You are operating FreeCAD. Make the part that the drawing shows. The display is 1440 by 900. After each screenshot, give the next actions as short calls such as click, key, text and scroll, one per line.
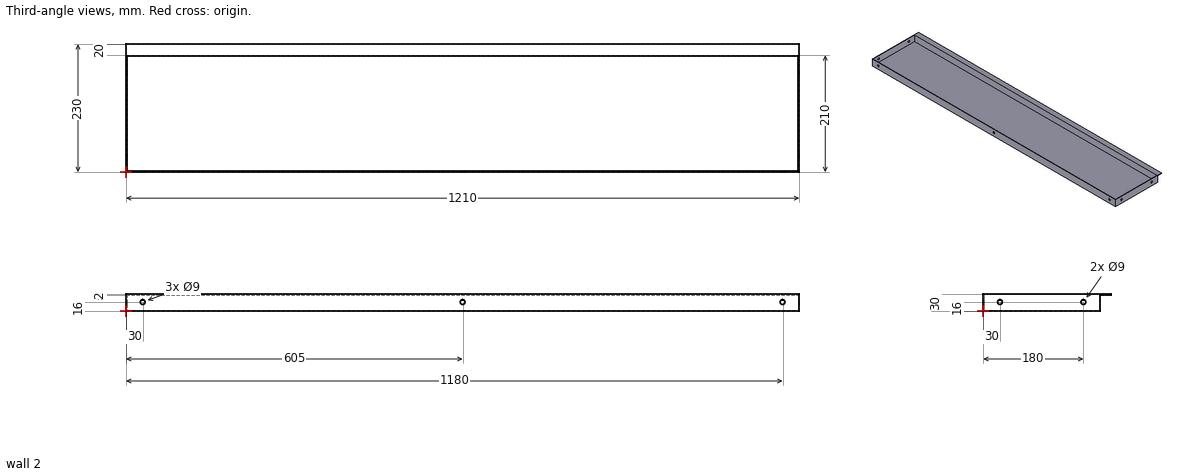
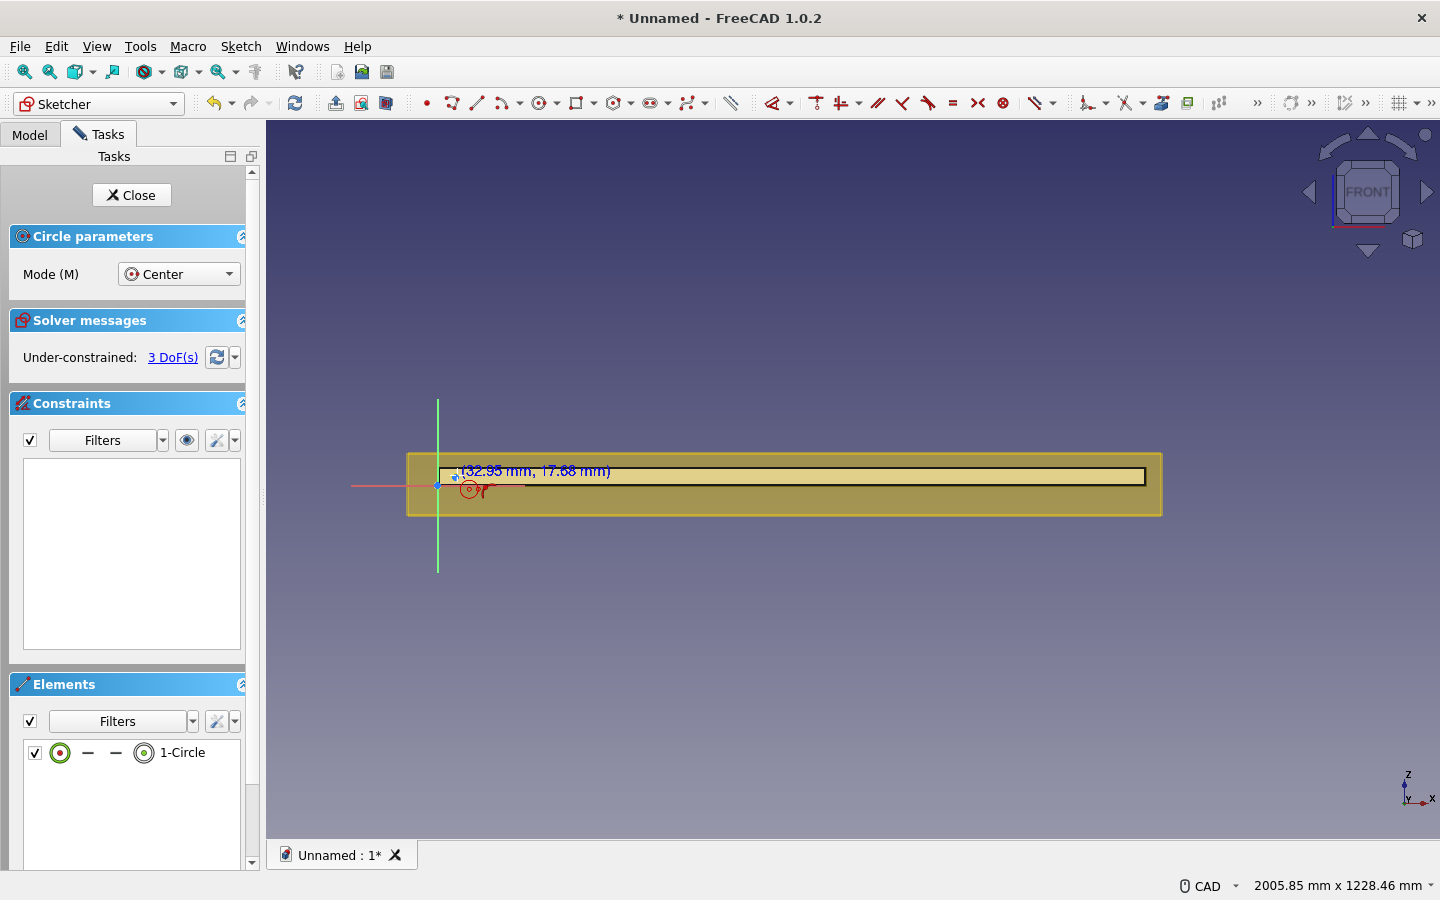
scroll(1128, 477, up, 11)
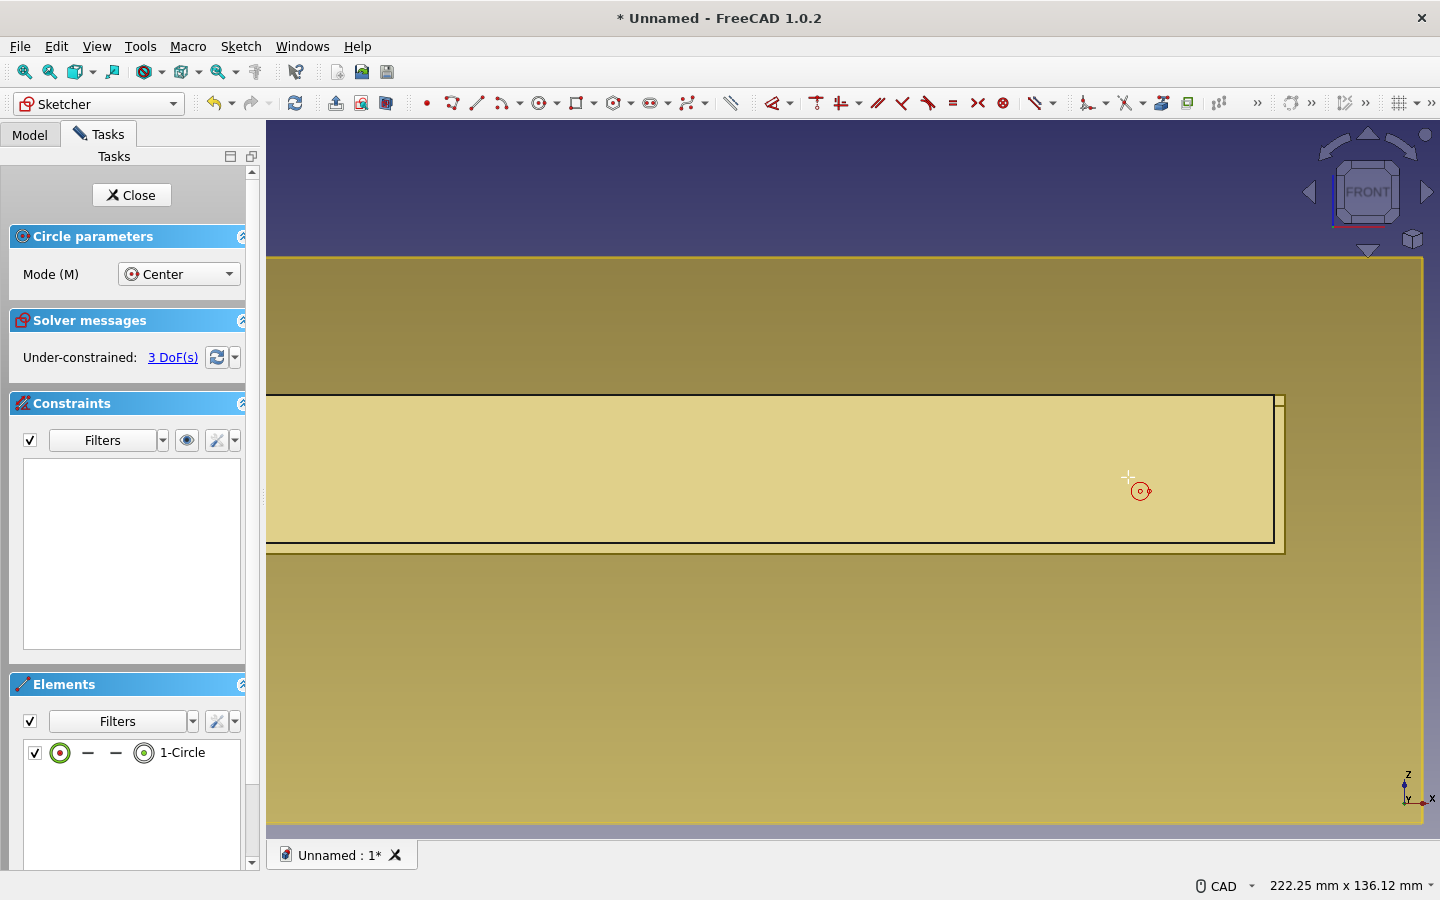
scroll(1129, 477, down, 11)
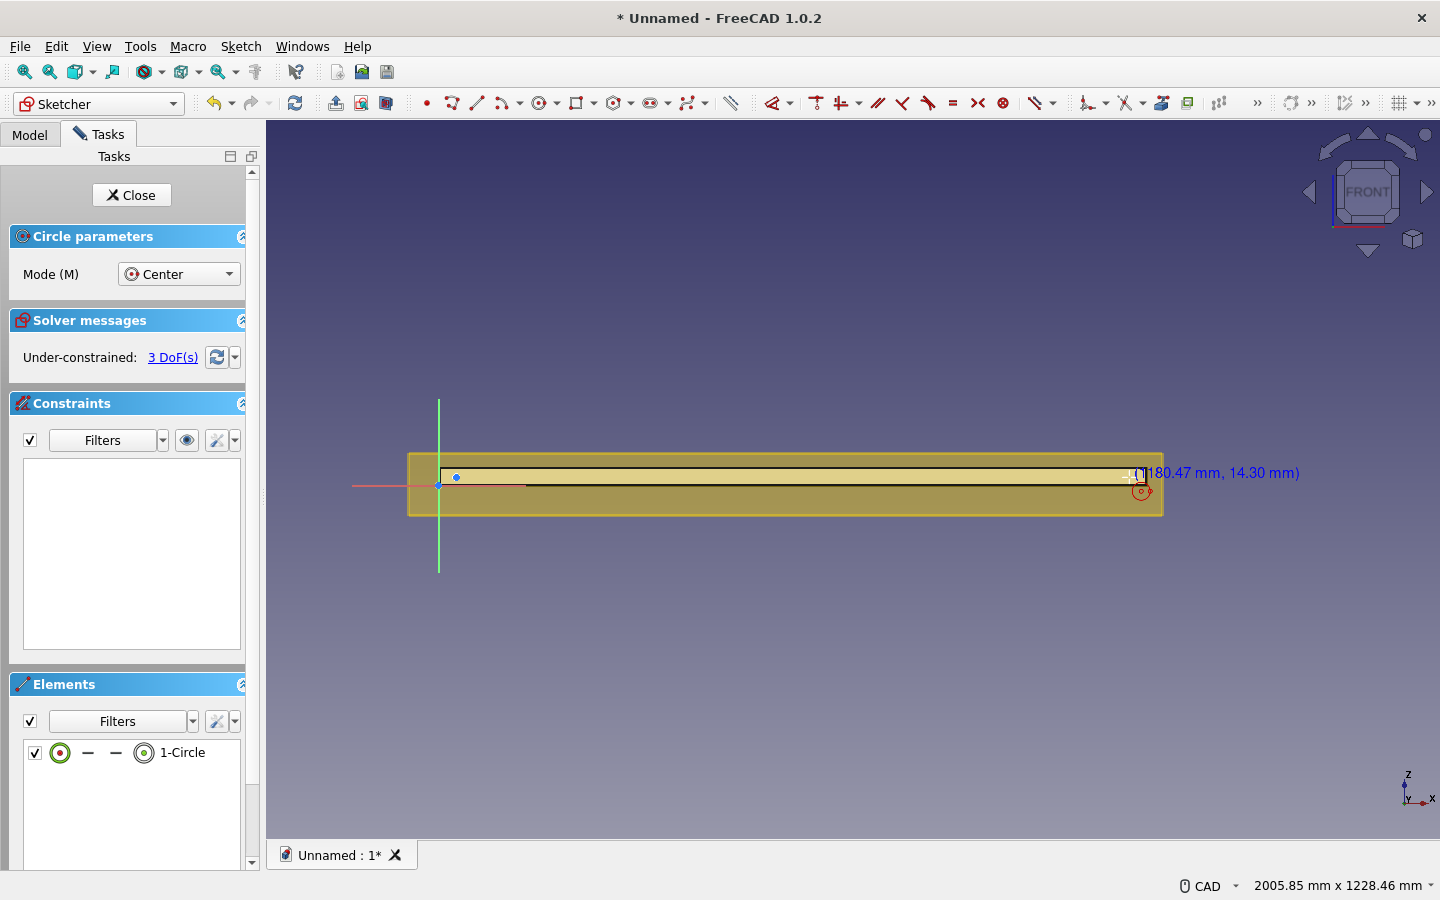
scroll(1129, 477, up, 3)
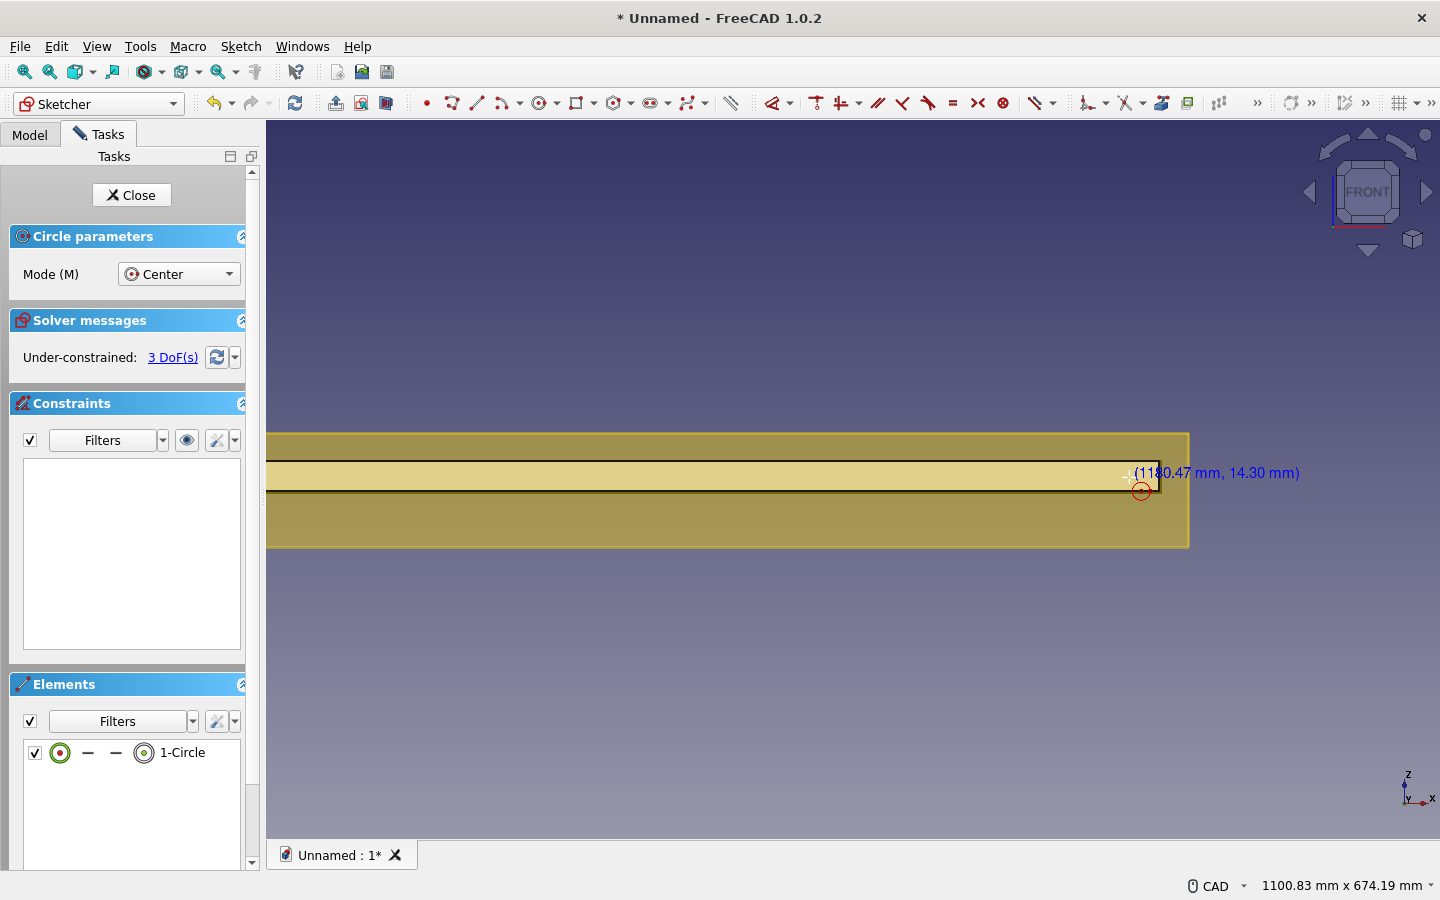
click(1129, 476)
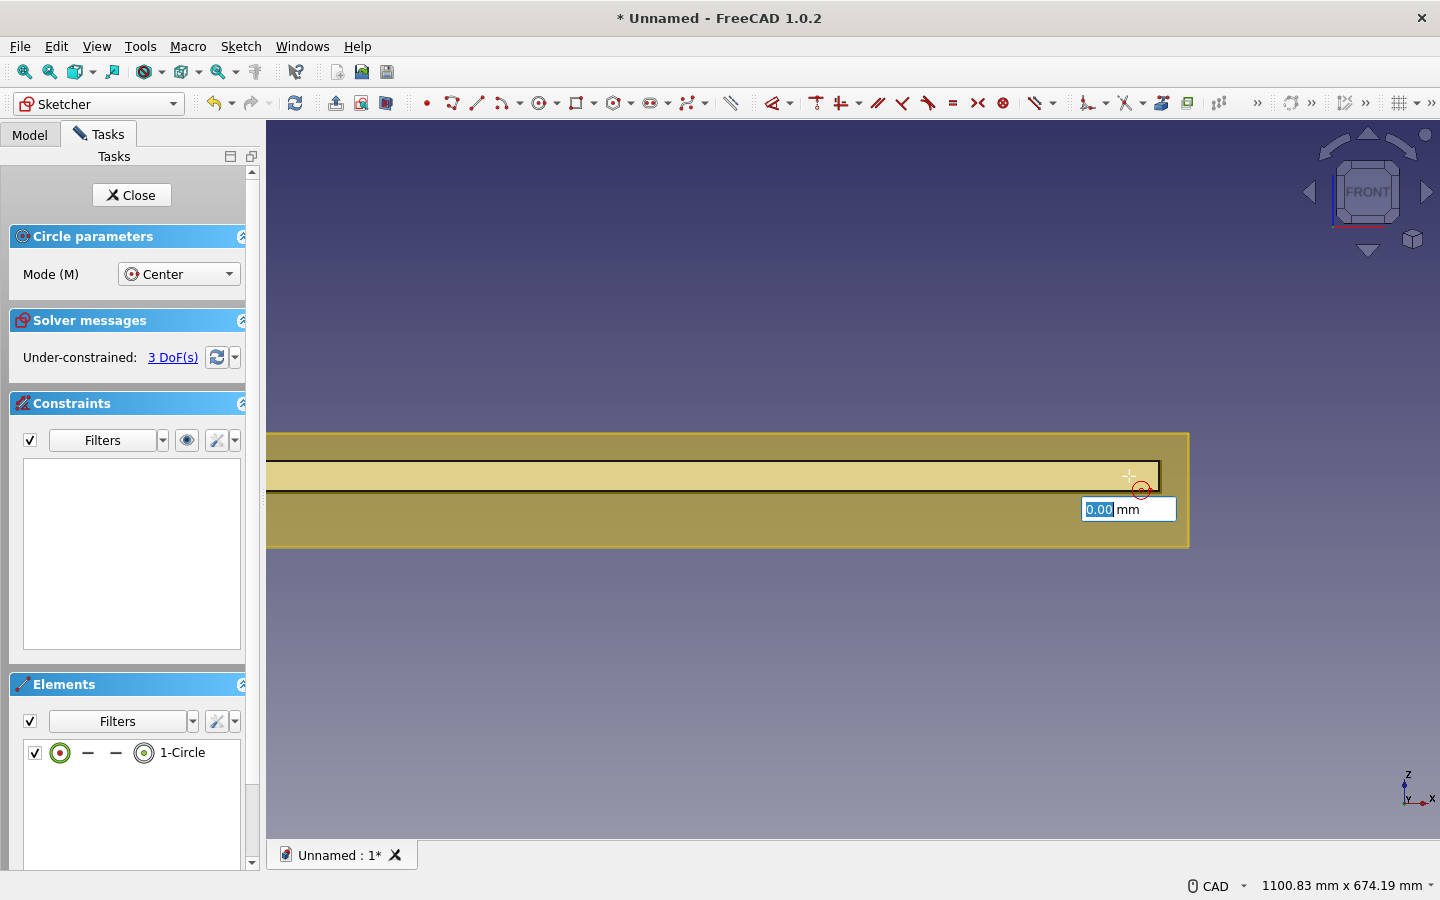
scroll(1132, 472, up, 6)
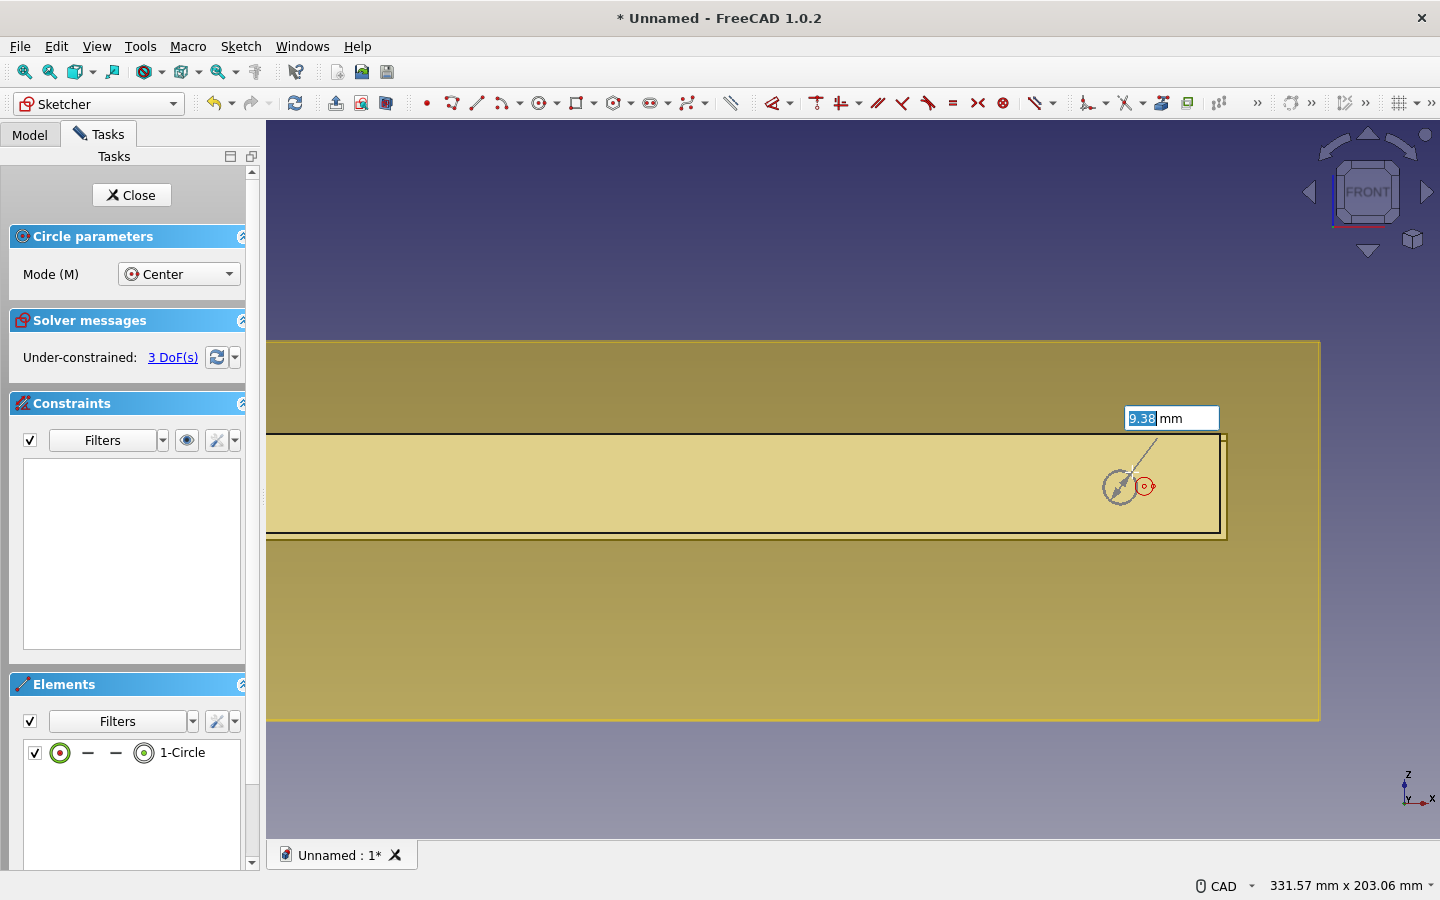
click(1132, 472)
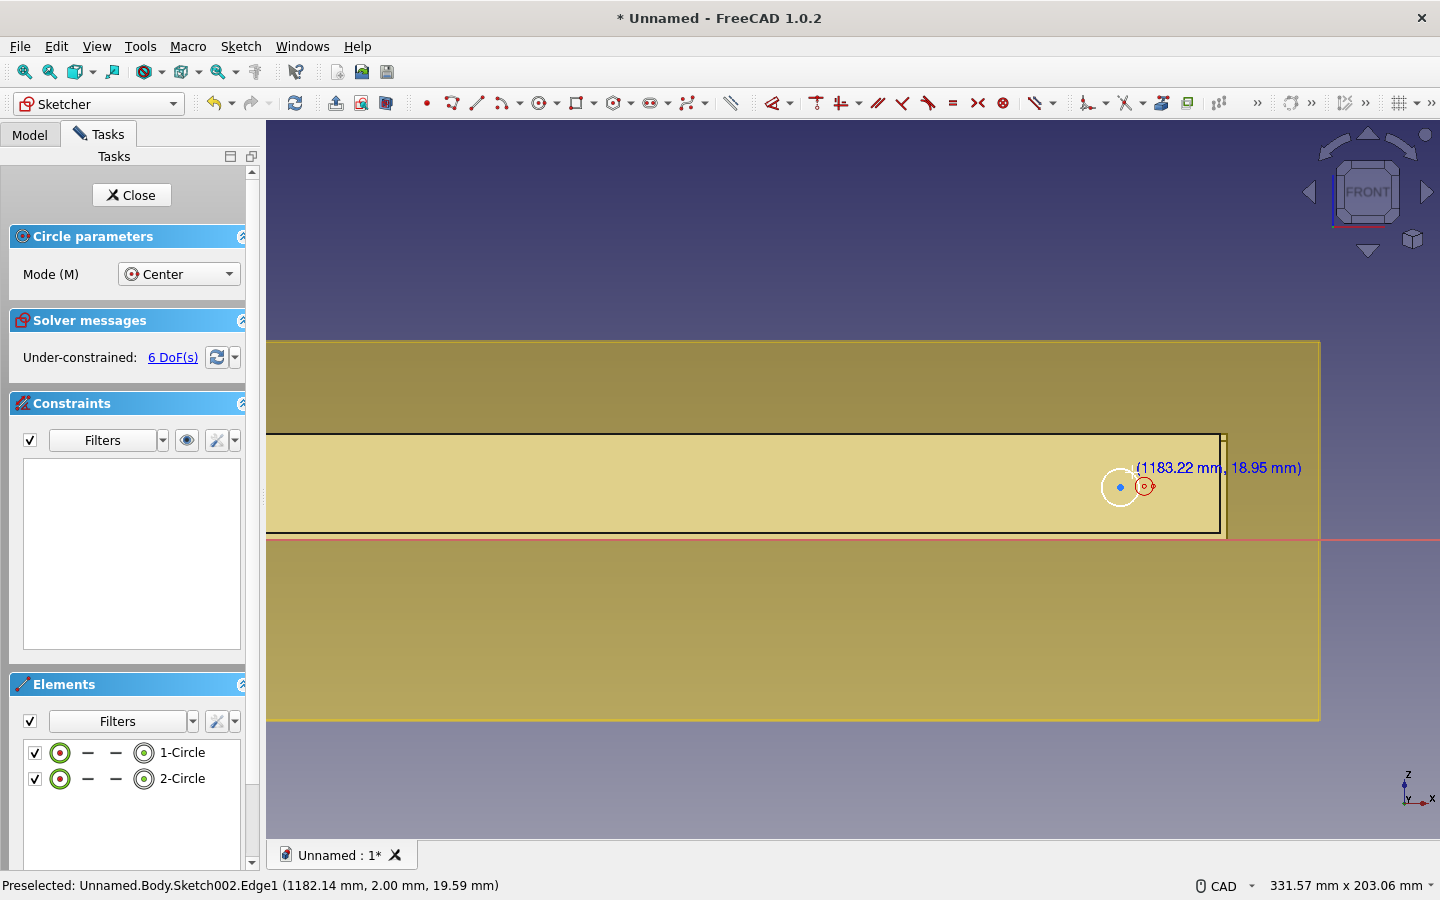
scroll(1130, 475, down, 9)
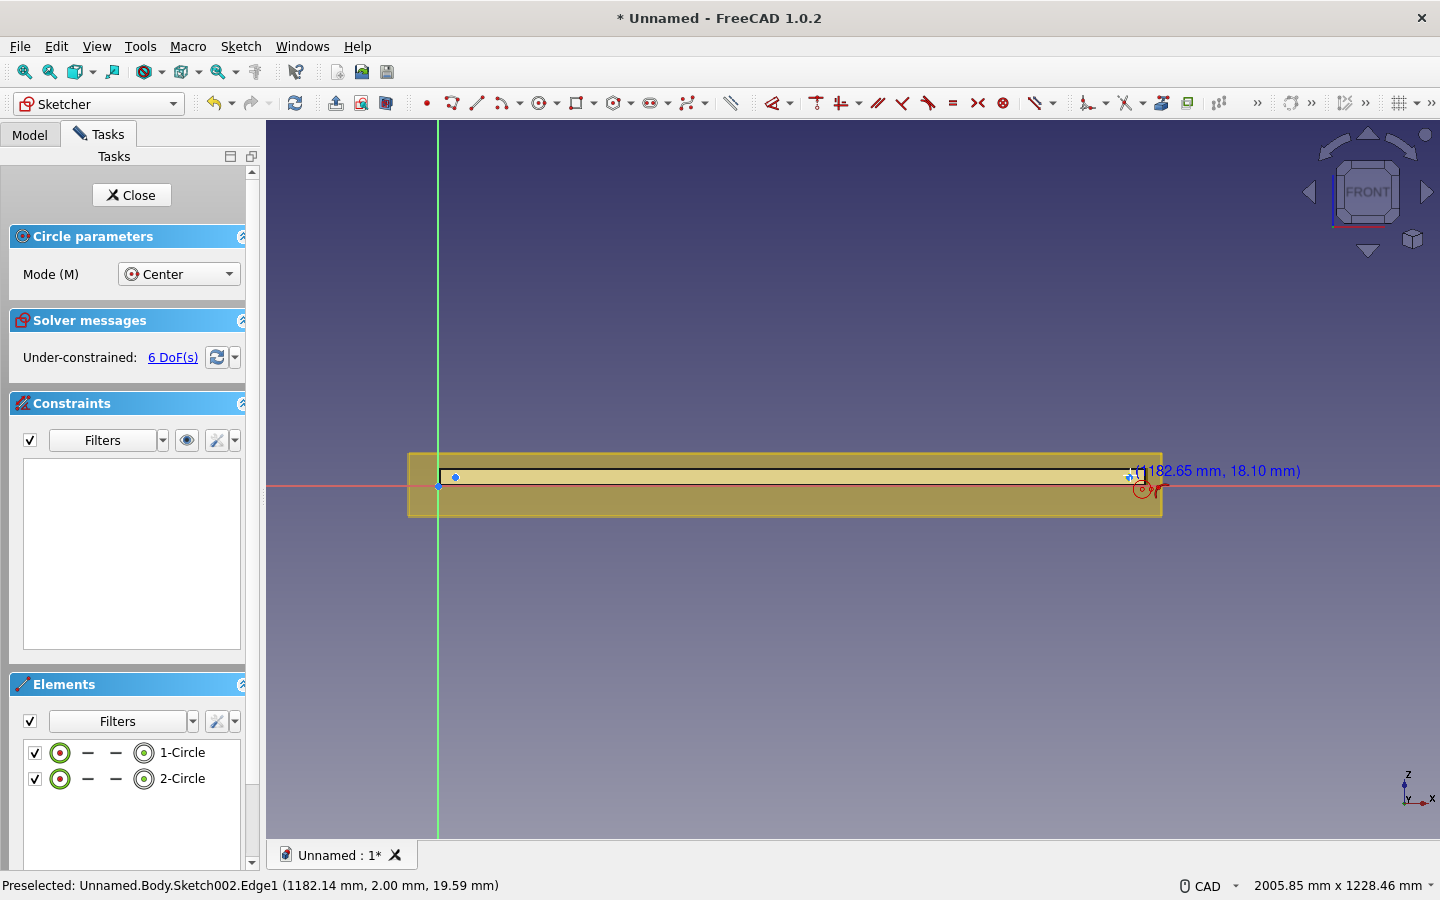
scroll(793, 477, up, 11)